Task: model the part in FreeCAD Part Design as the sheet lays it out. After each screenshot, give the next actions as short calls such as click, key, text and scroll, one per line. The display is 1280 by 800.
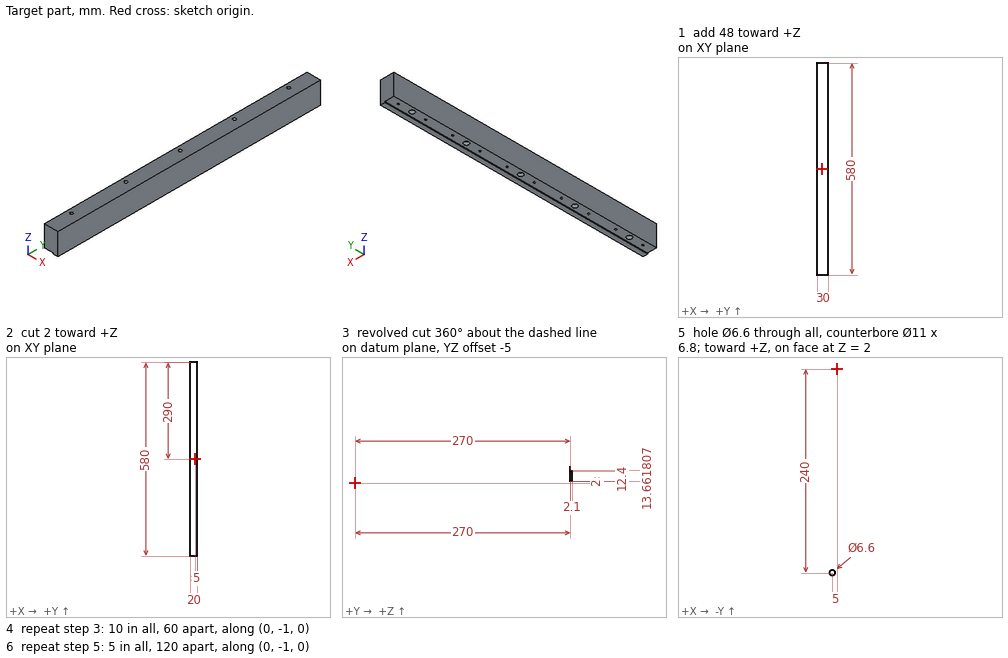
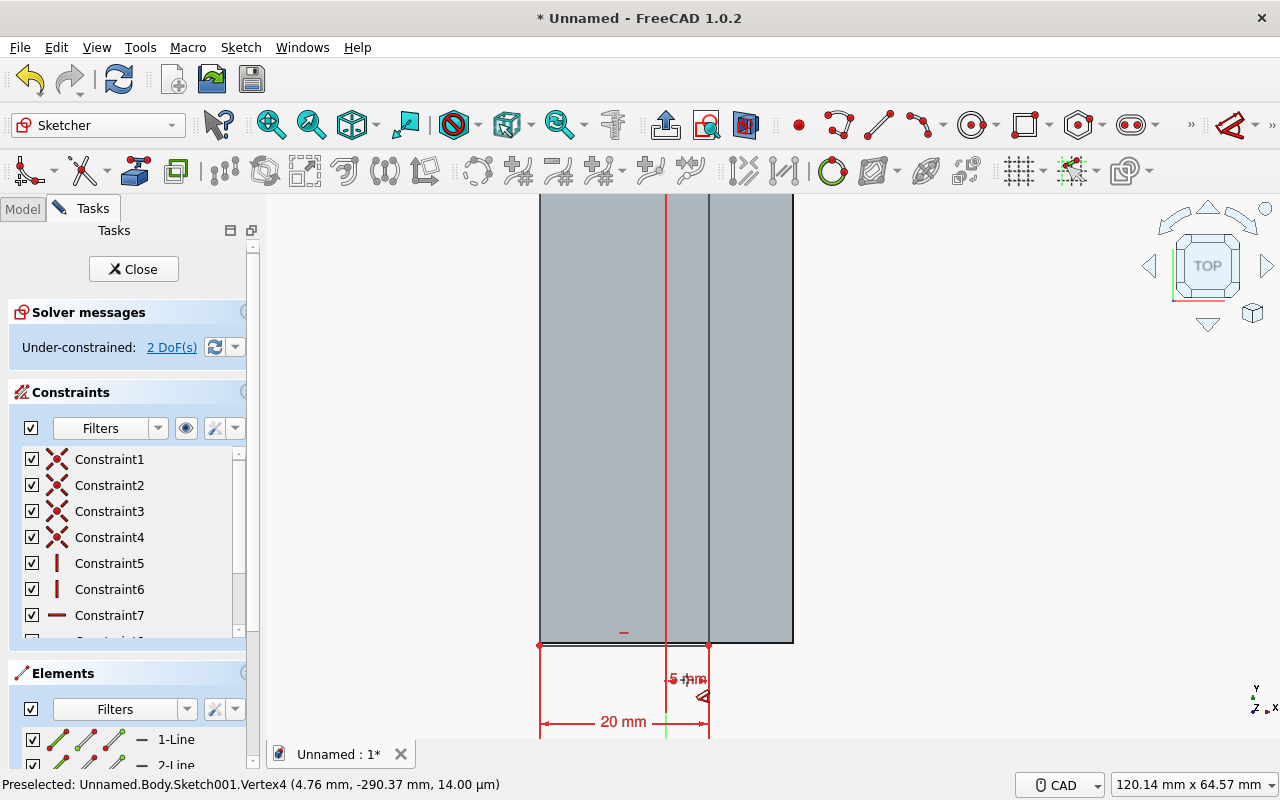
scroll(711, 649, down, 13)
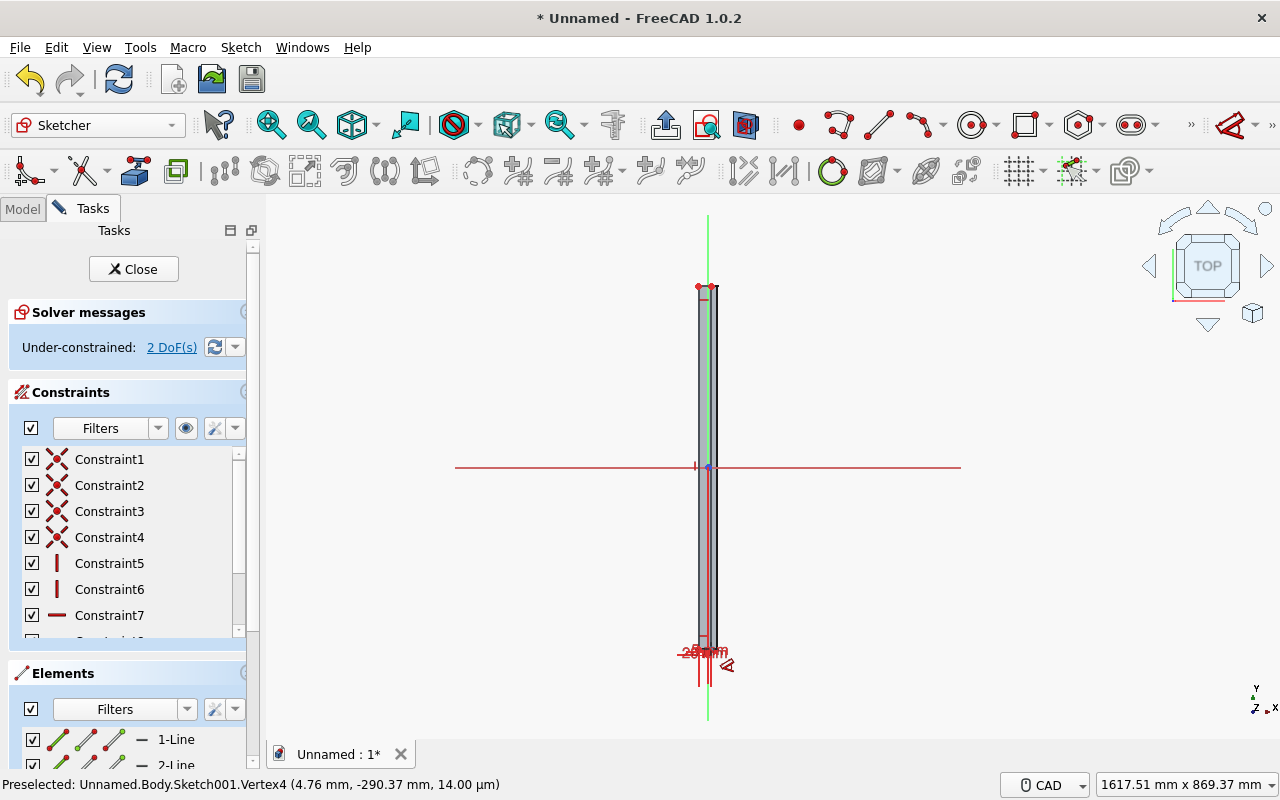
scroll(699, 395, up, 2)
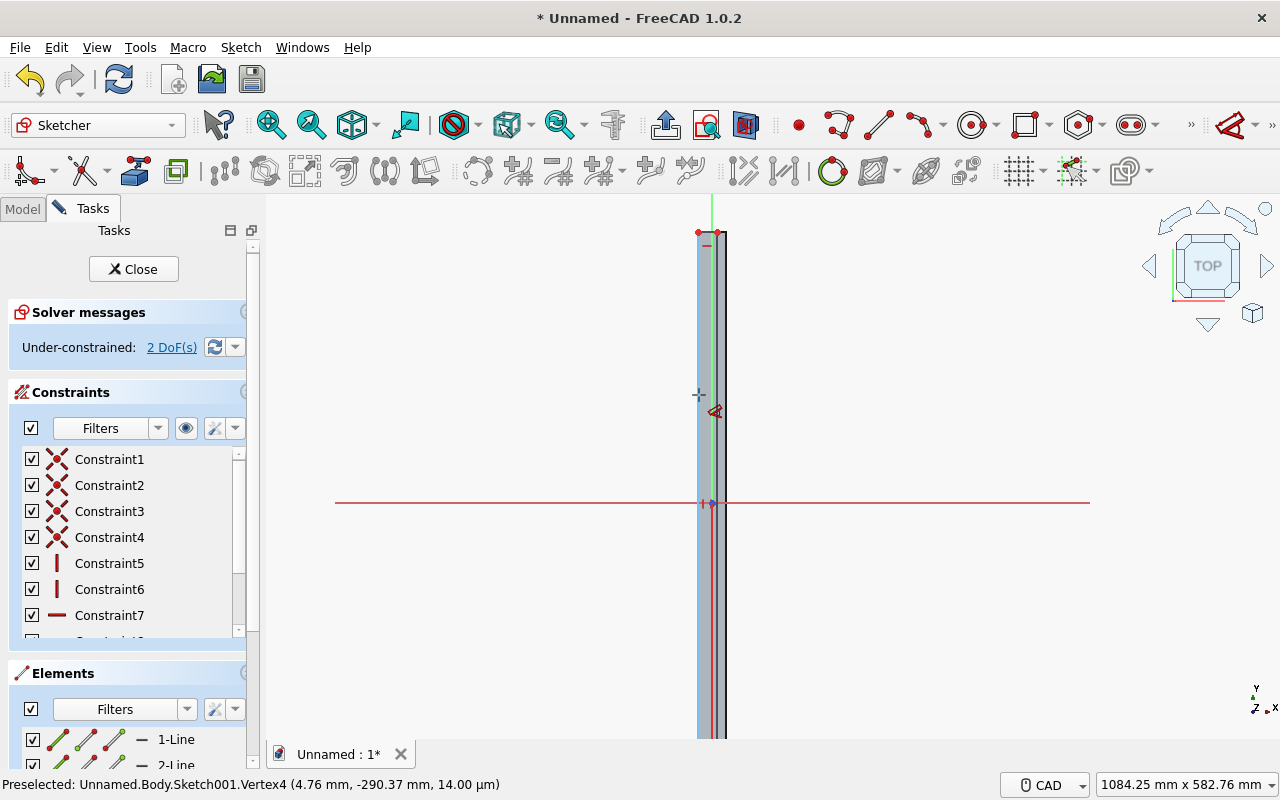
click(698, 395)
click(664, 472)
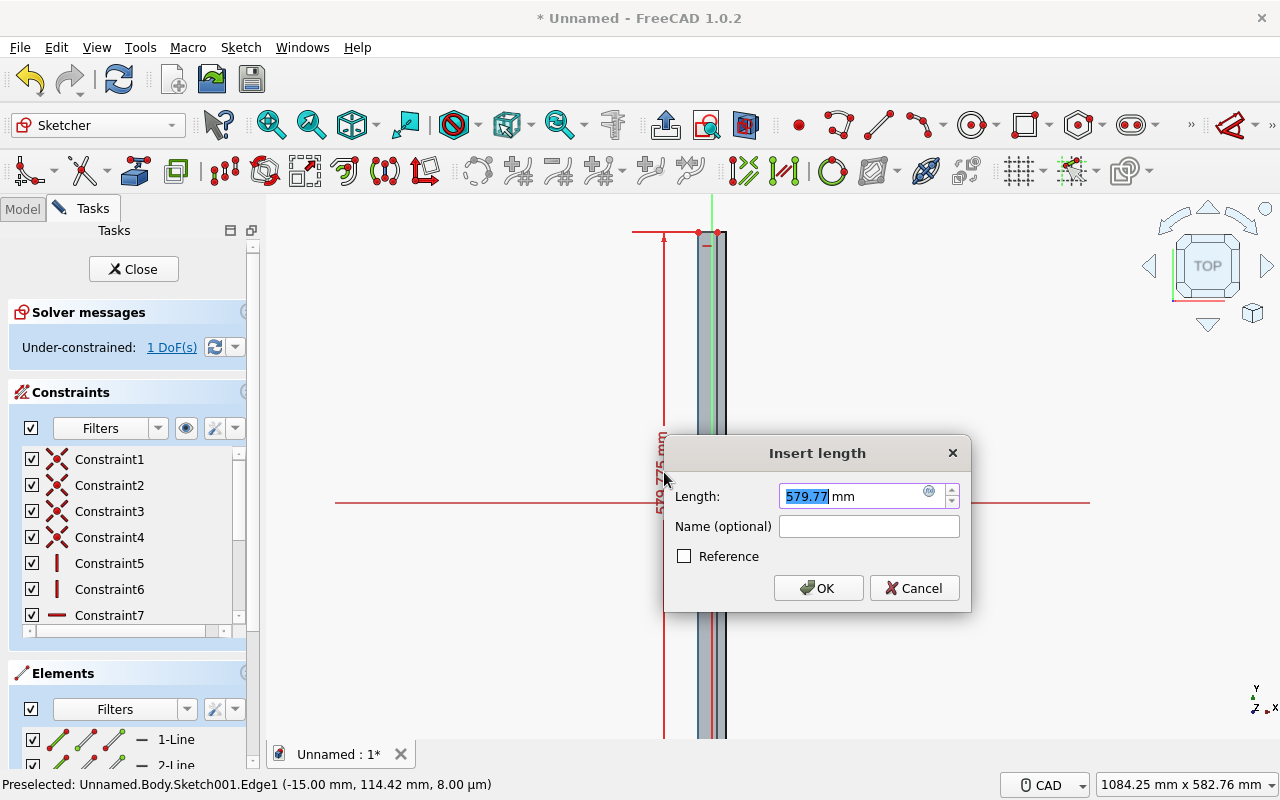
text(580)
key(Return)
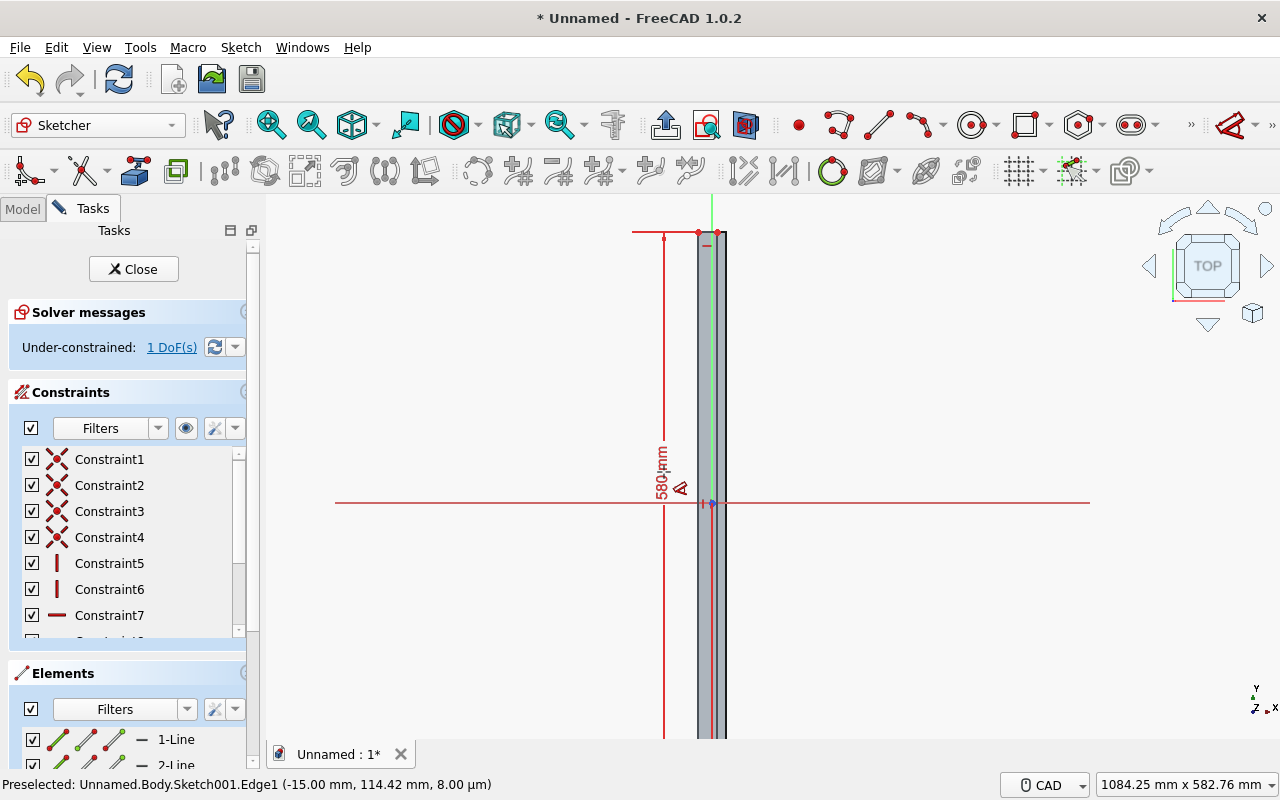
click(698, 232)
click(664, 368)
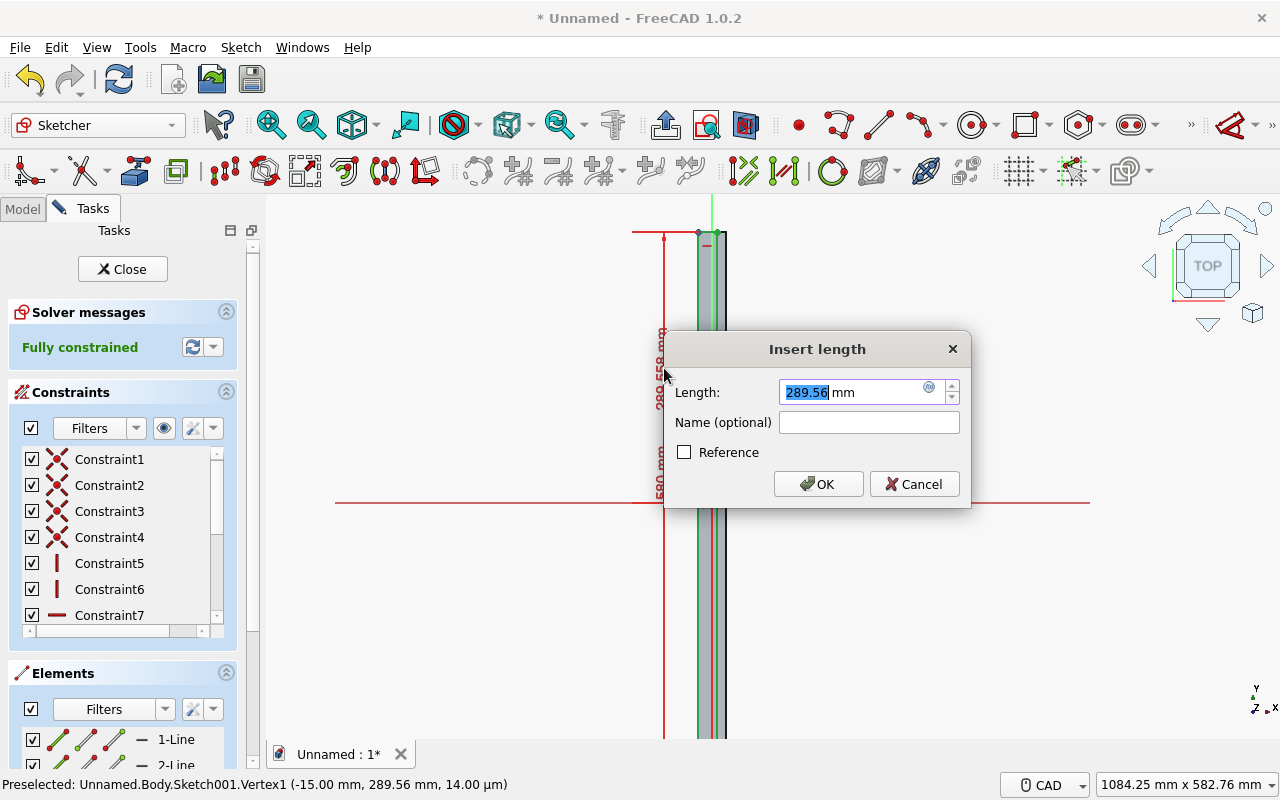
text(290)
key(Return)
key(Escape)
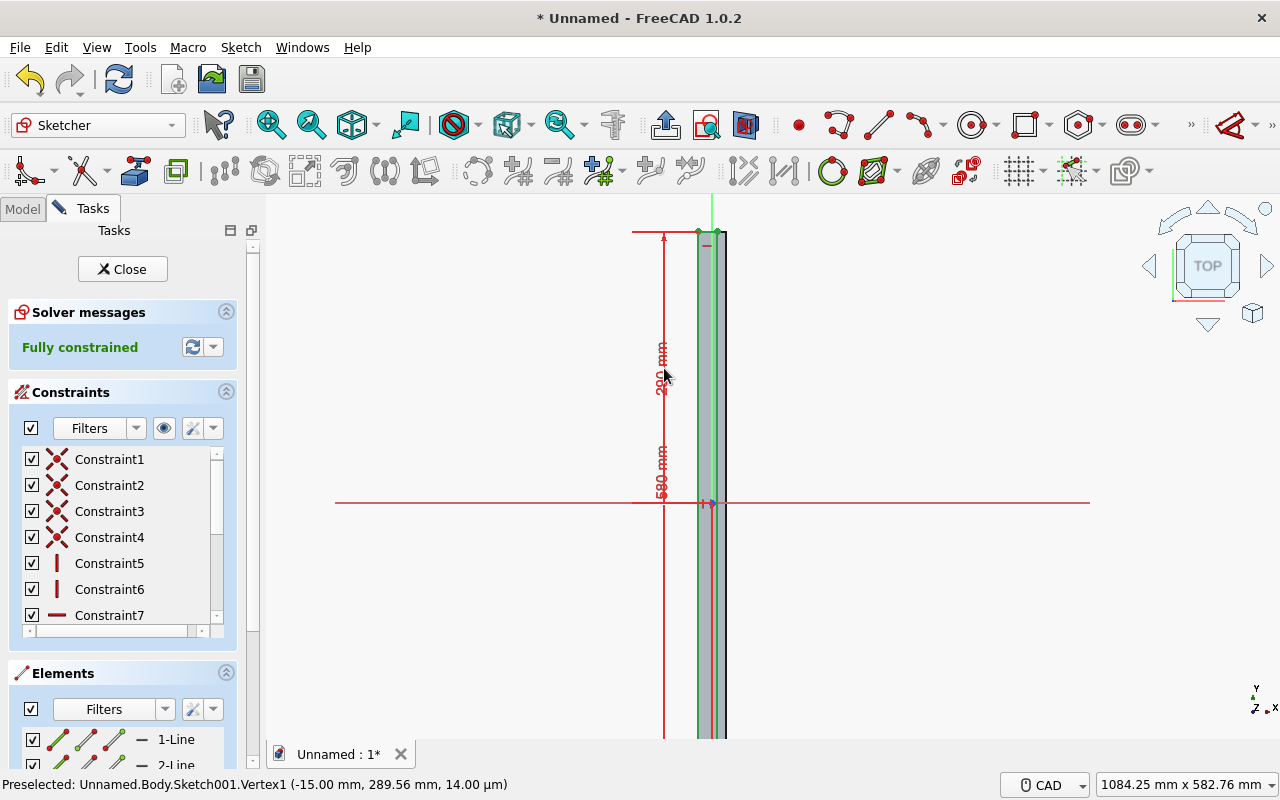
click(123, 269)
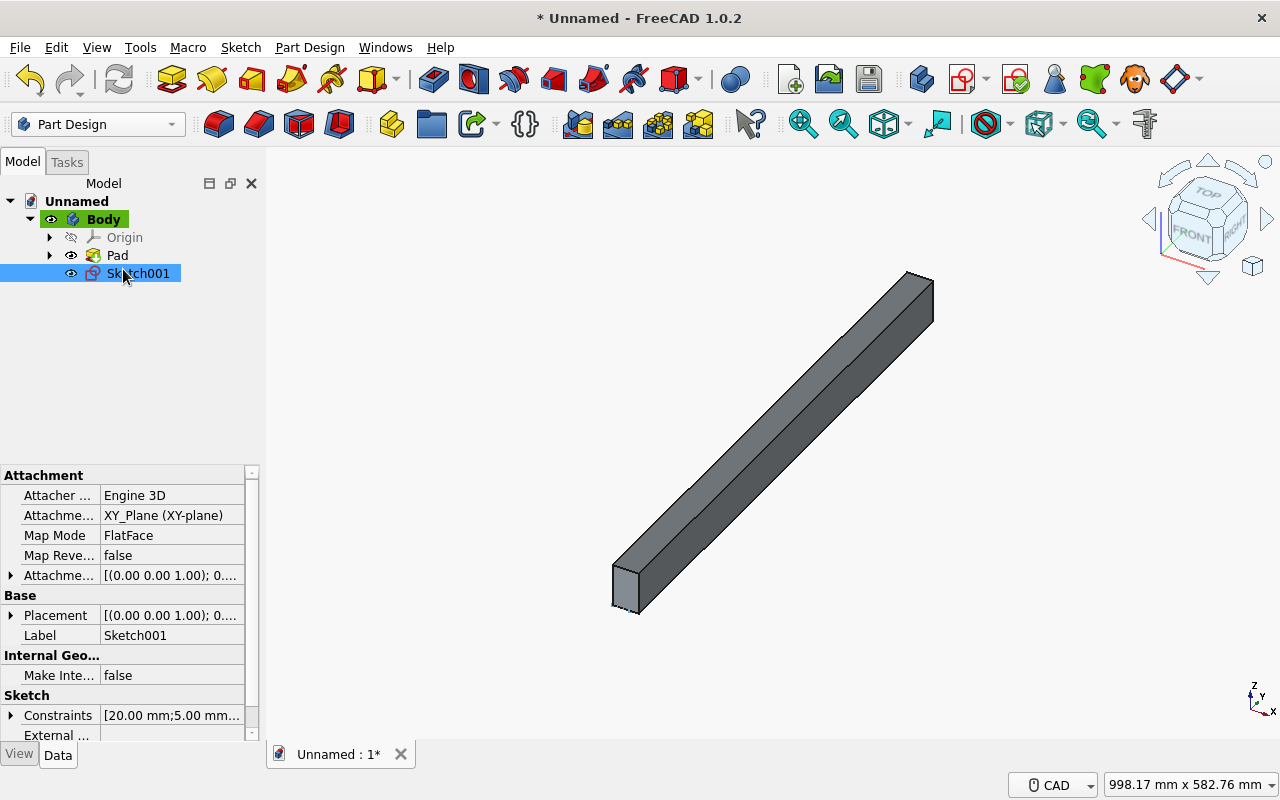
click(434, 80)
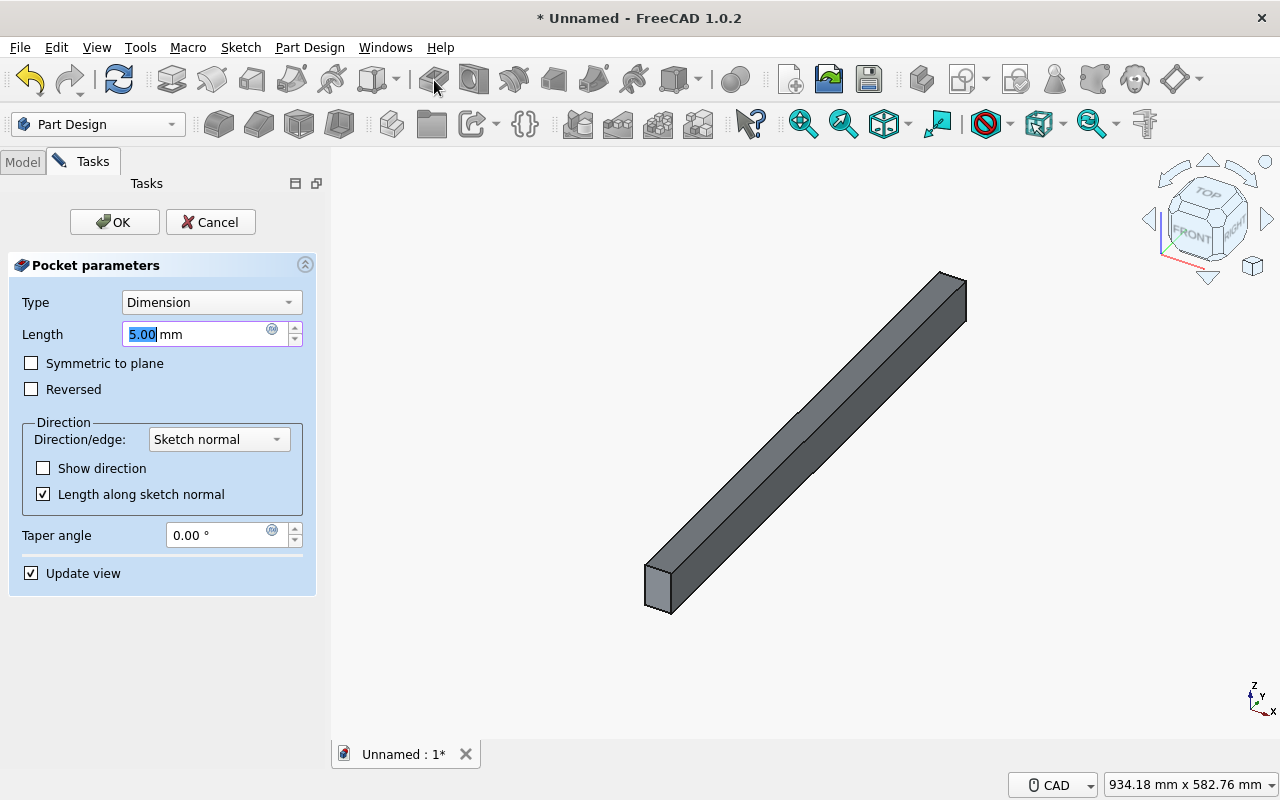
text(2)
key(Tab)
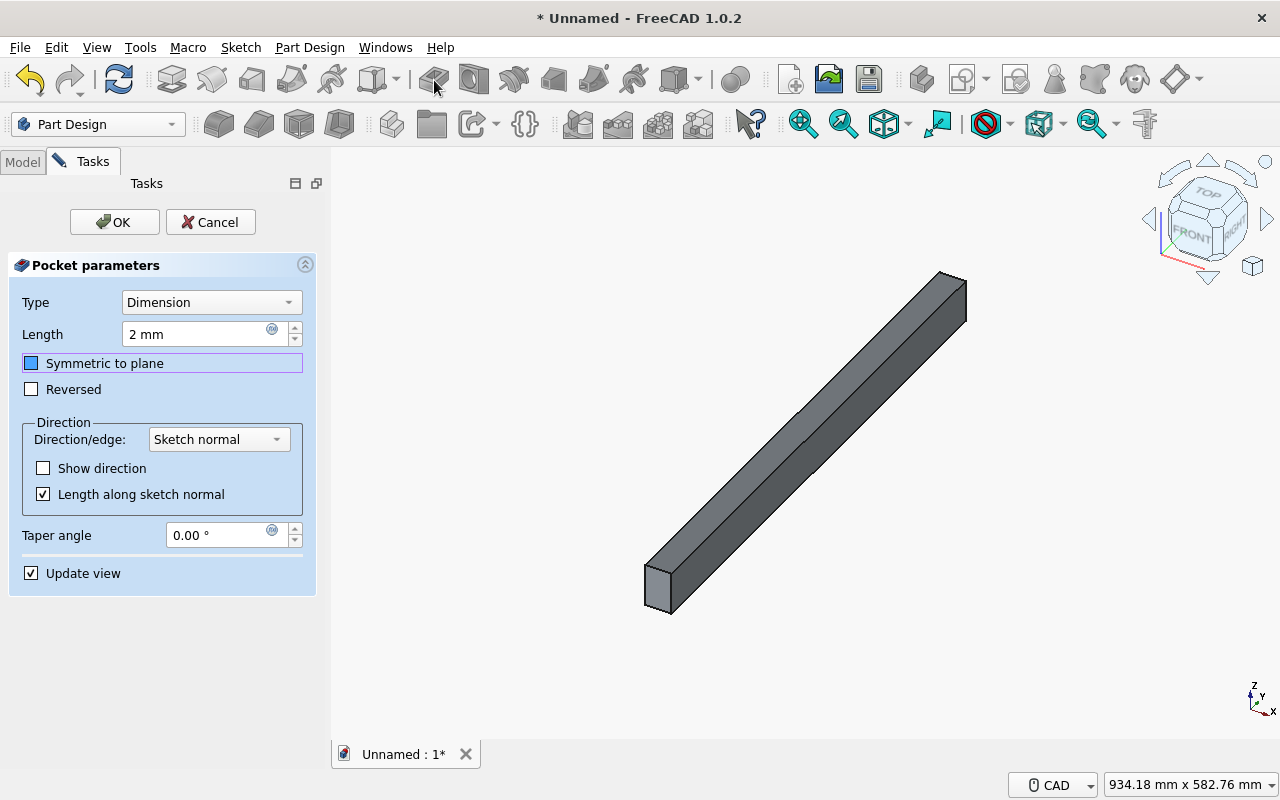
click(30, 389)